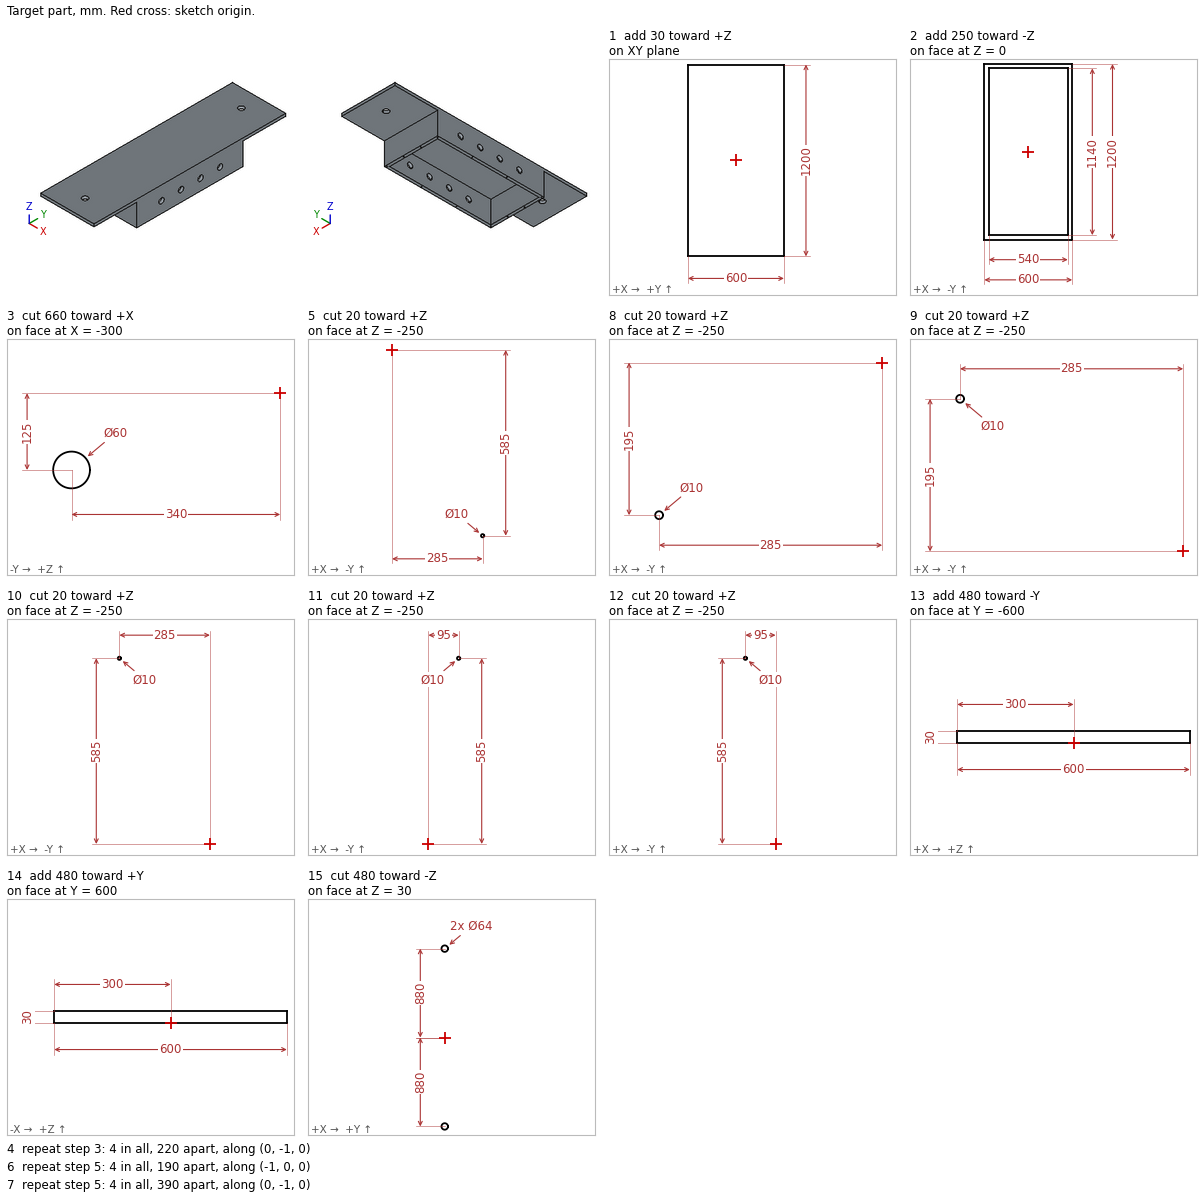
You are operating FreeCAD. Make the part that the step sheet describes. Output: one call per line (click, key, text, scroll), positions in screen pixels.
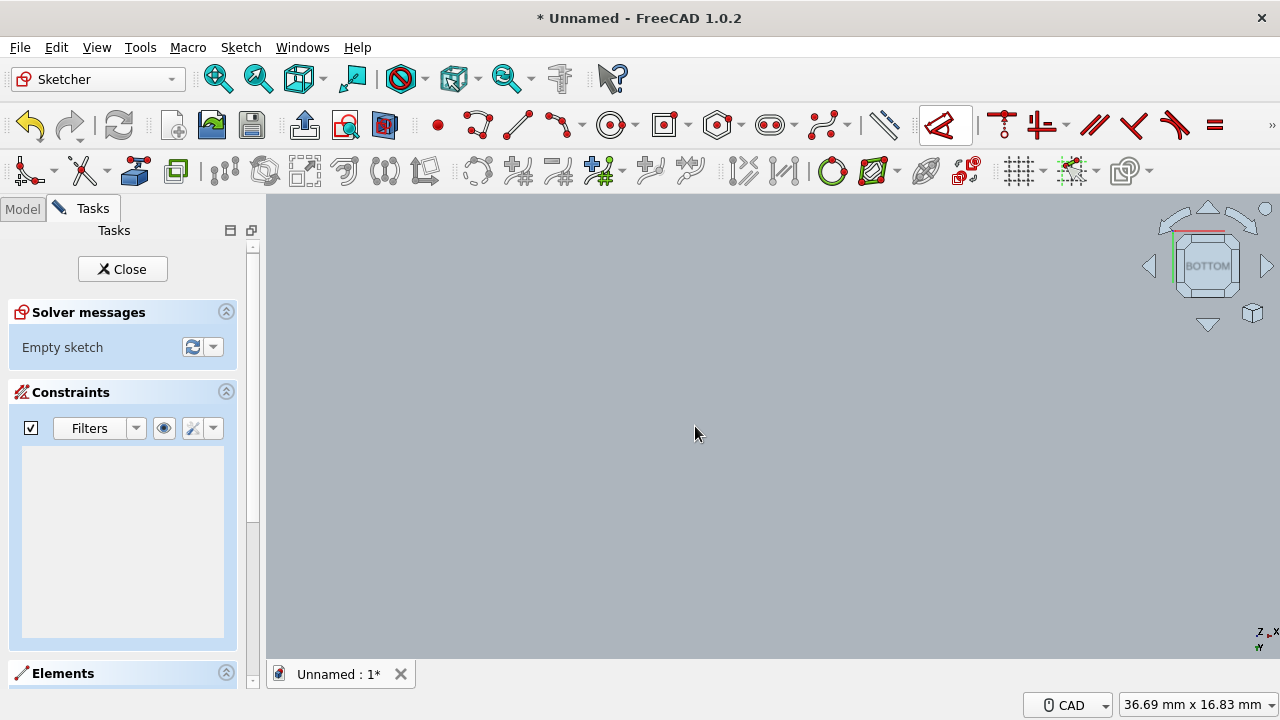
click(612, 126)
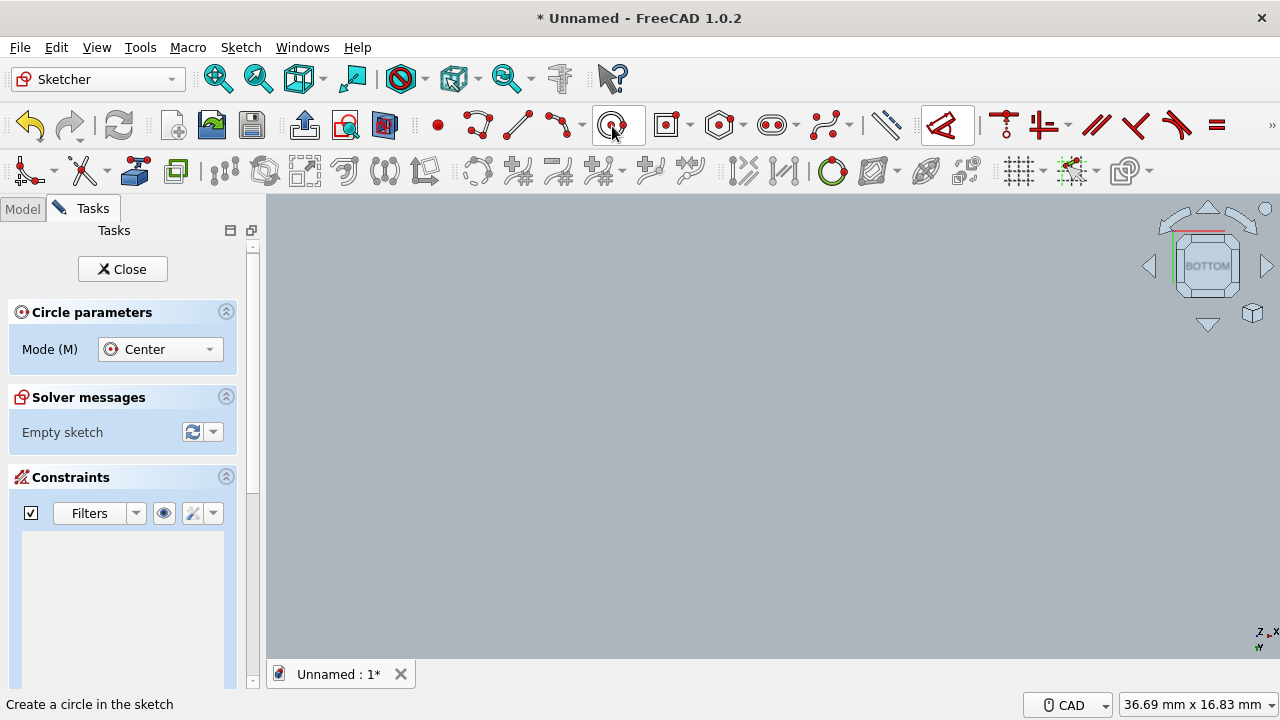
click(701, 424)
move(799, 327)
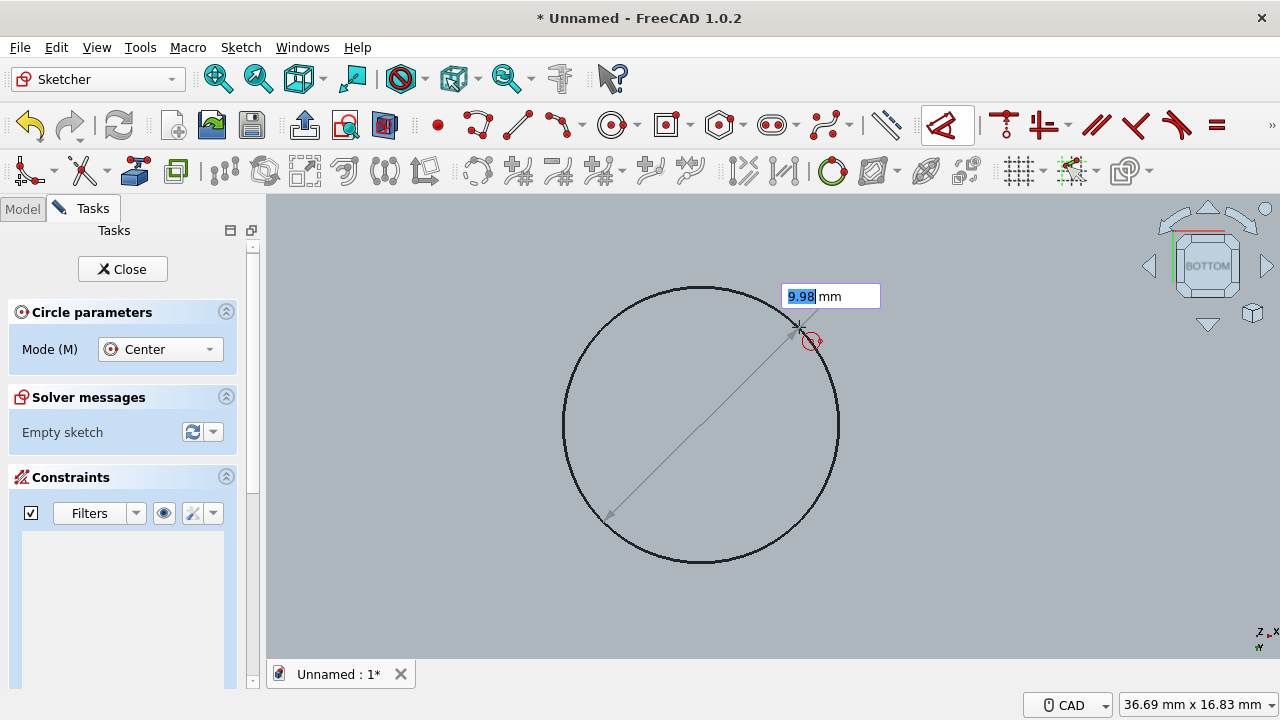
text(10)
key(Return)
key(Escape)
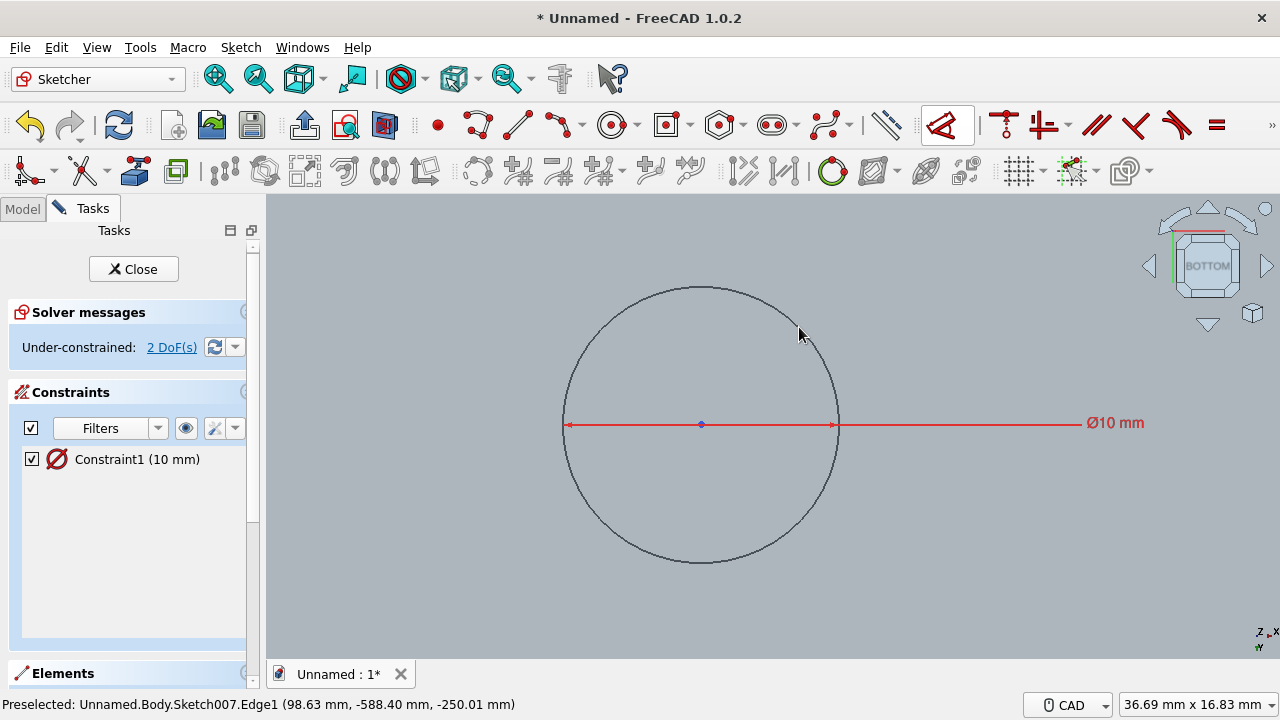
click(701, 425)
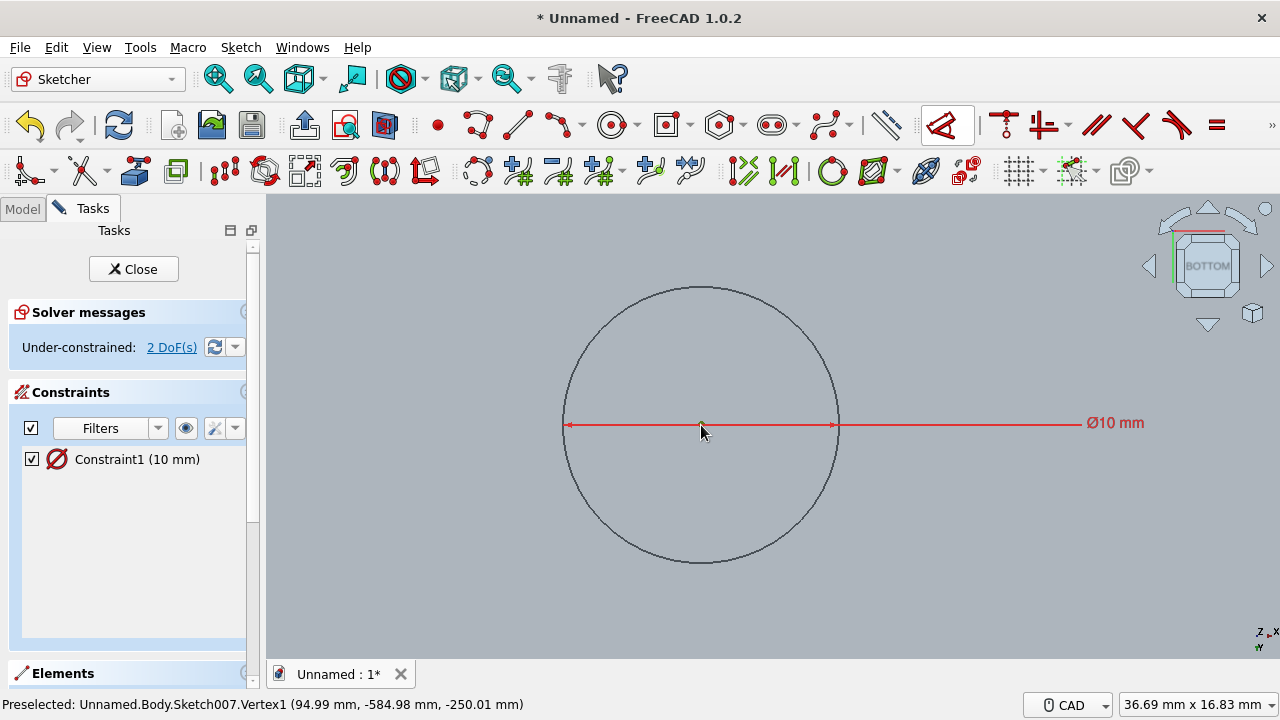
key(l)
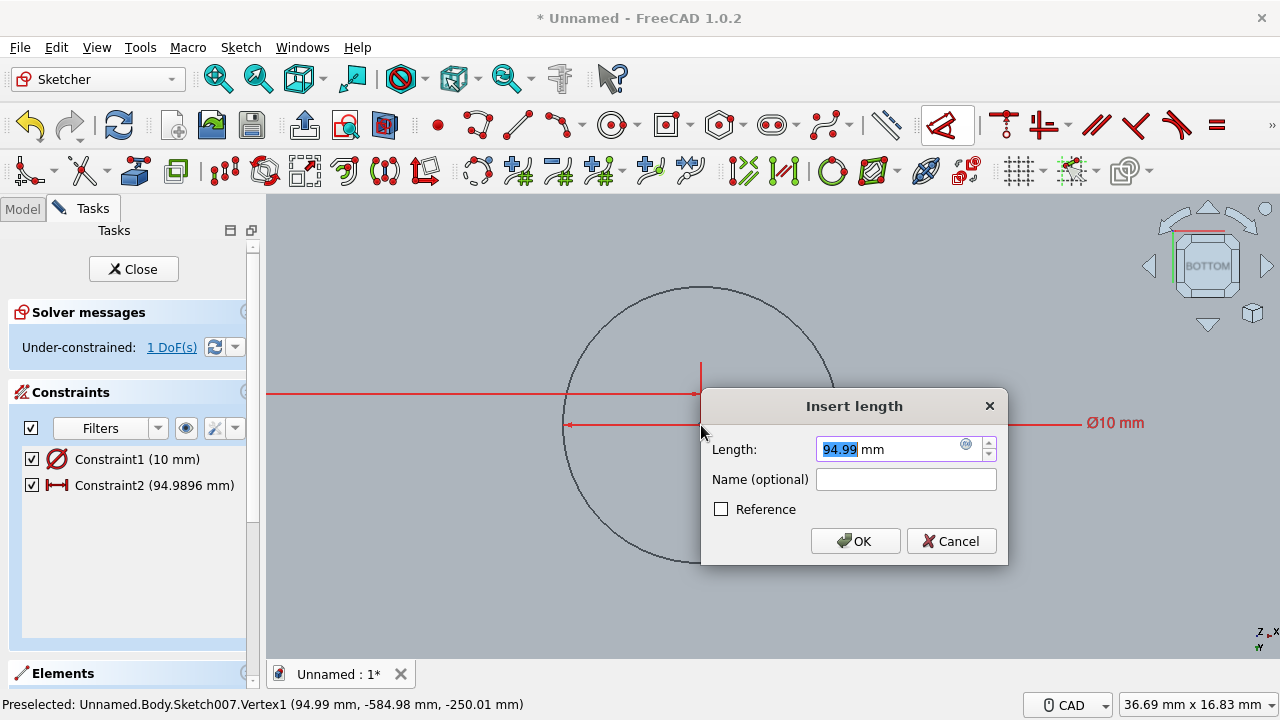
text(95)
key(Return)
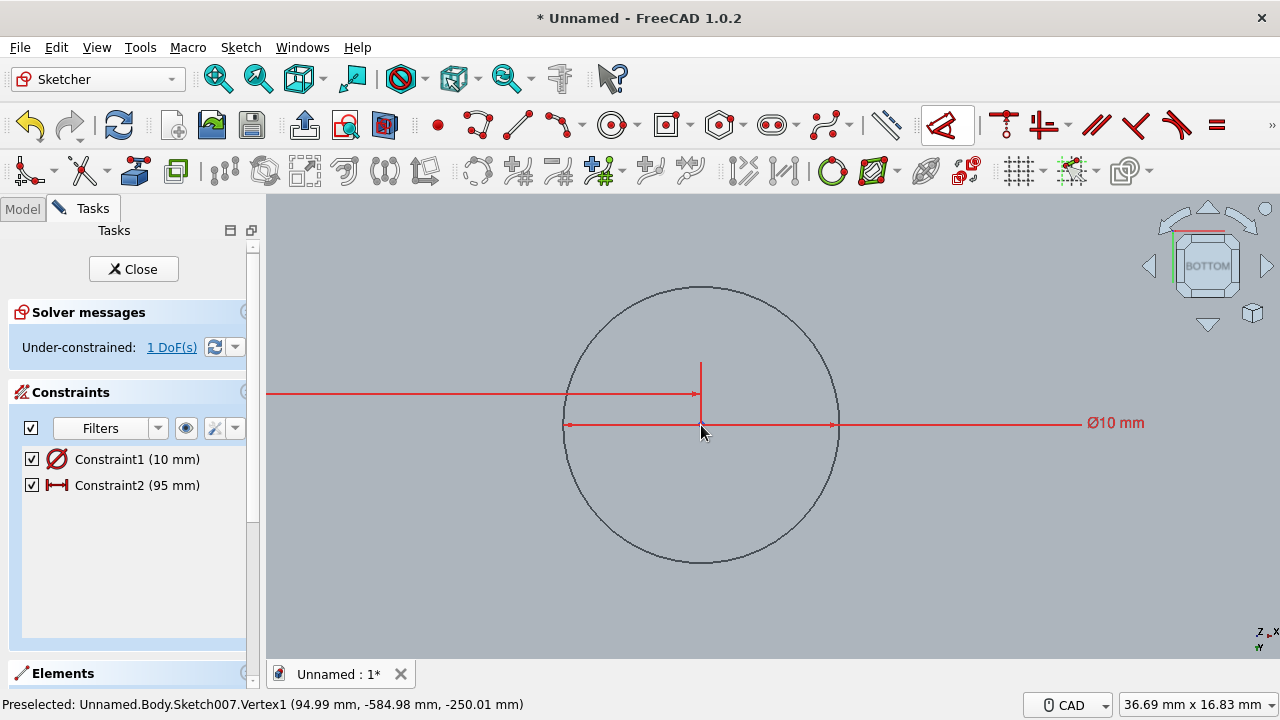
click(701, 425)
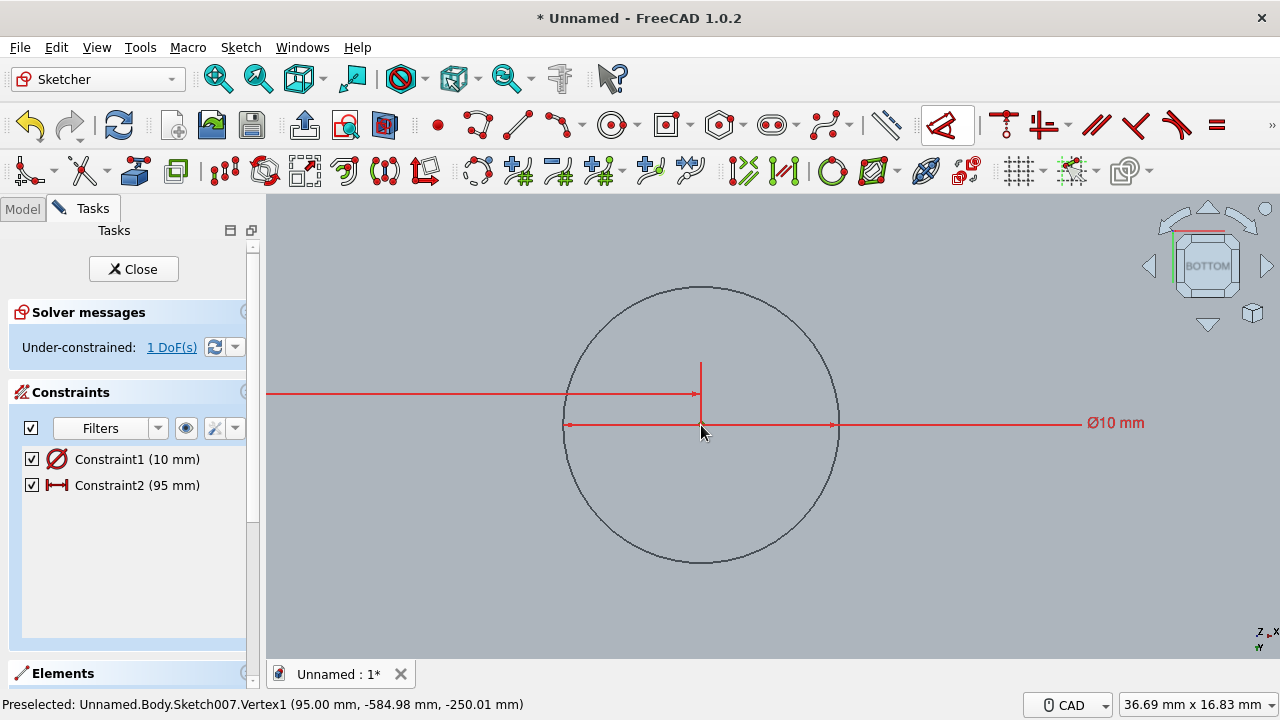
key(i)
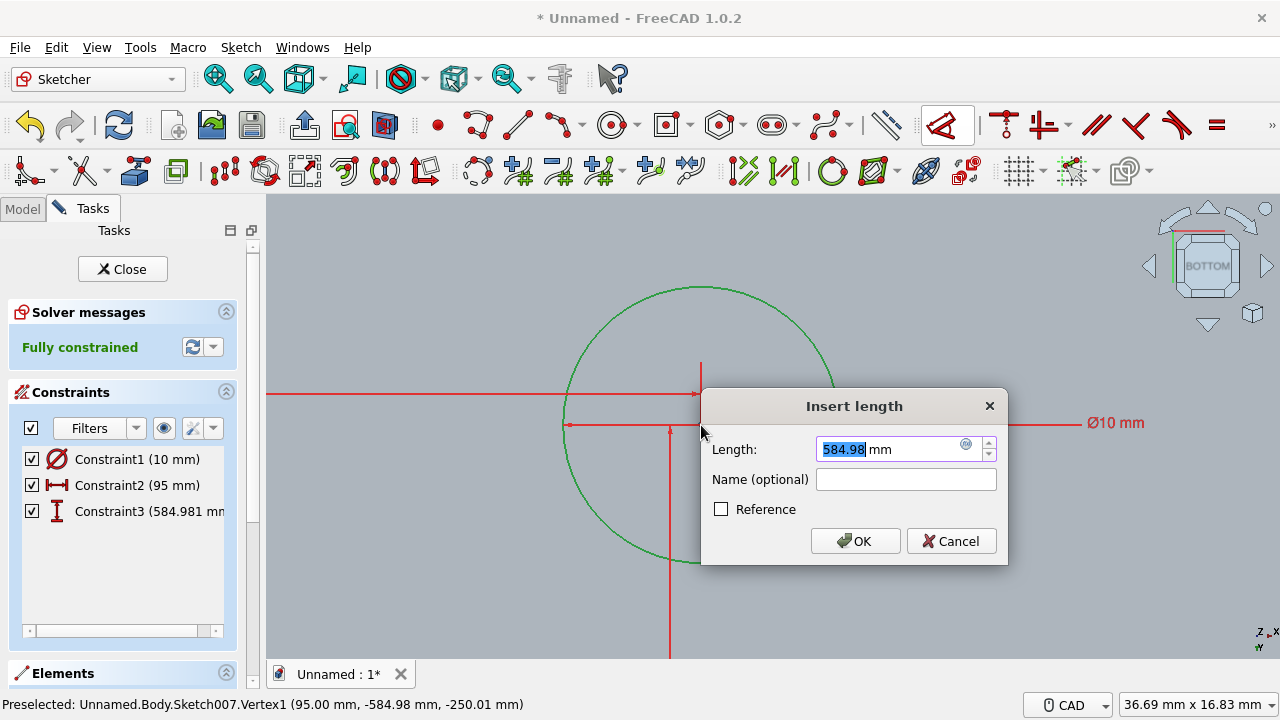
text(585)
key(Return)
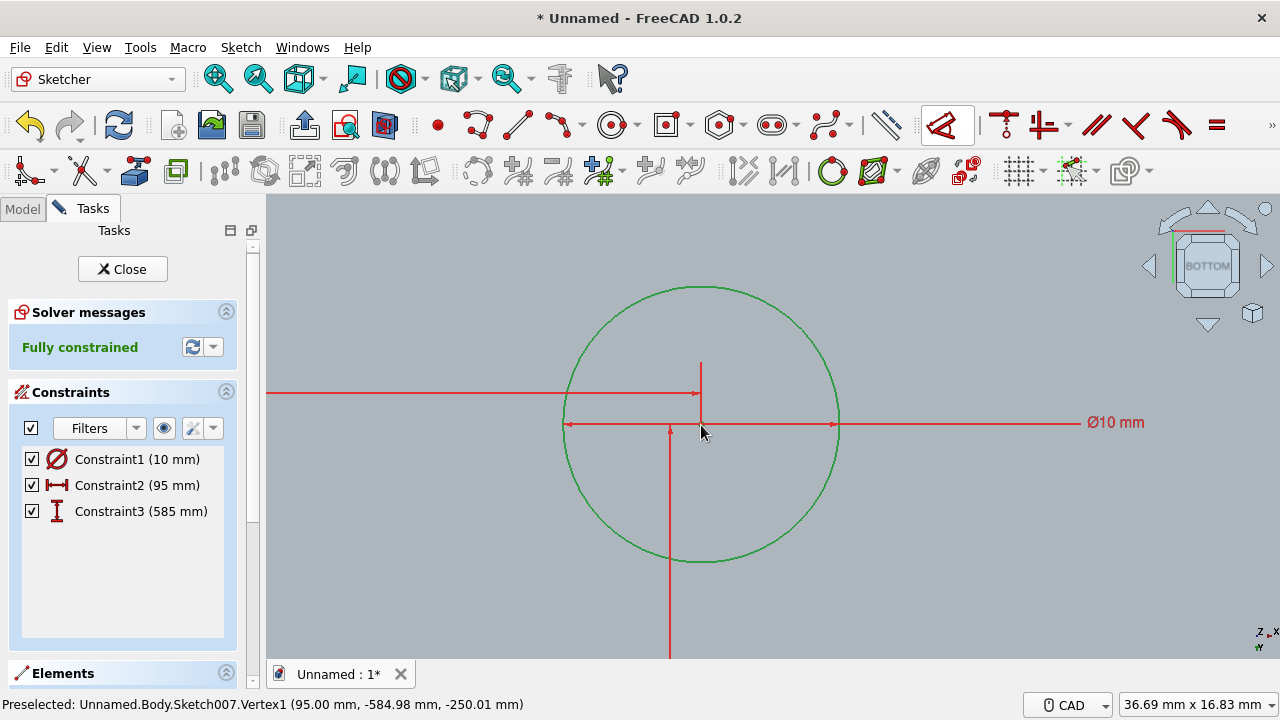
click(123, 269)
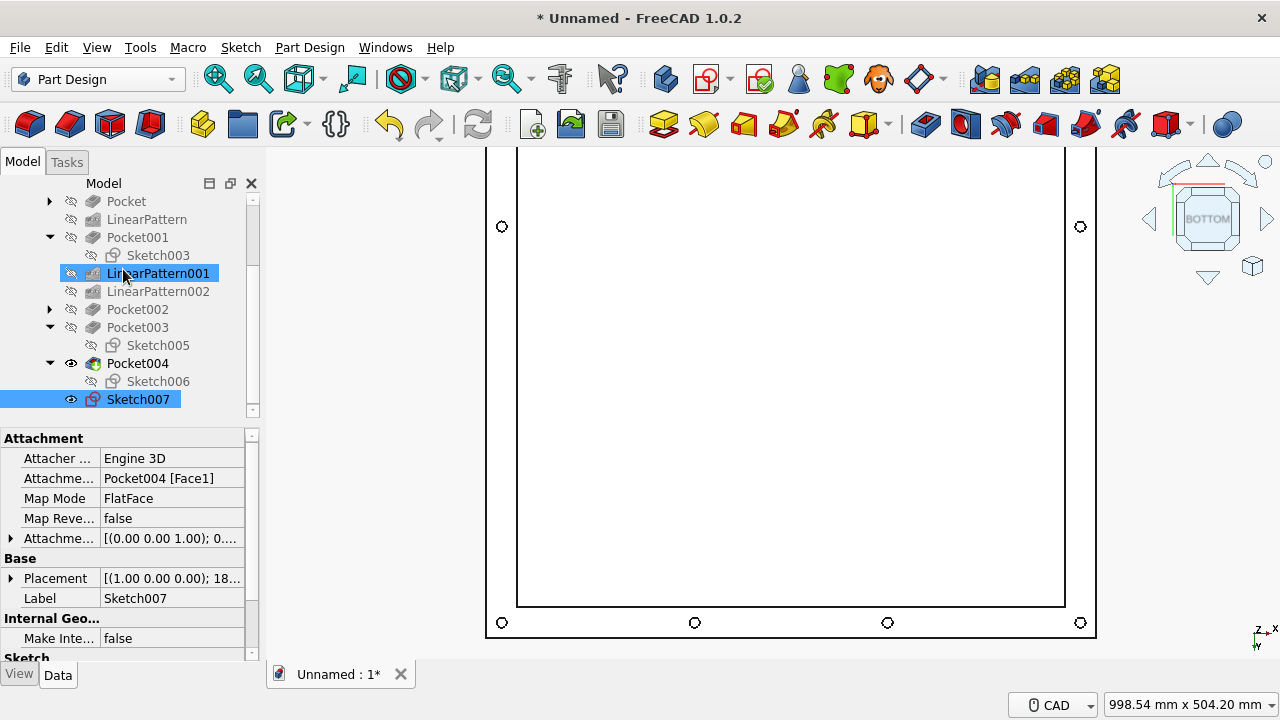
click(926, 124)